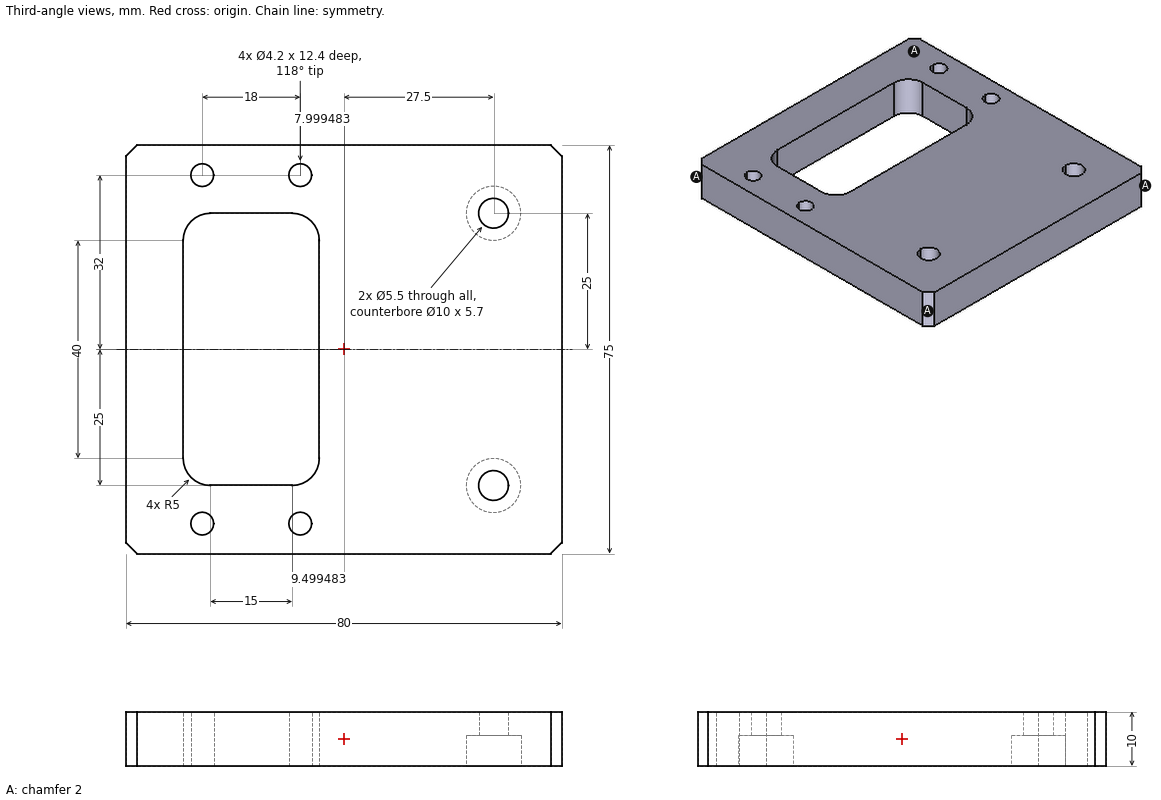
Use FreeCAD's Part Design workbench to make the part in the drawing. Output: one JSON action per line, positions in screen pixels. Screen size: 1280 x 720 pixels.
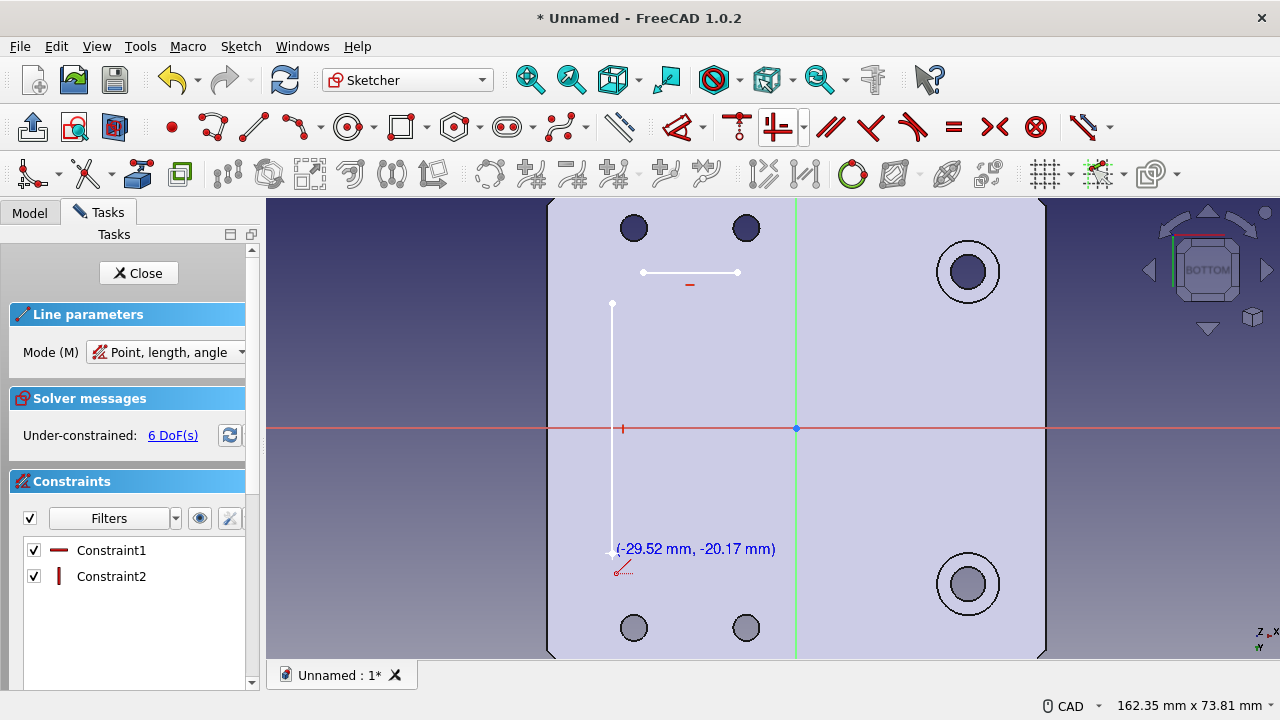
{"action": "left_click", "coordinate": [643, 584]}
{"action": "left_click", "coordinate": [737, 584]}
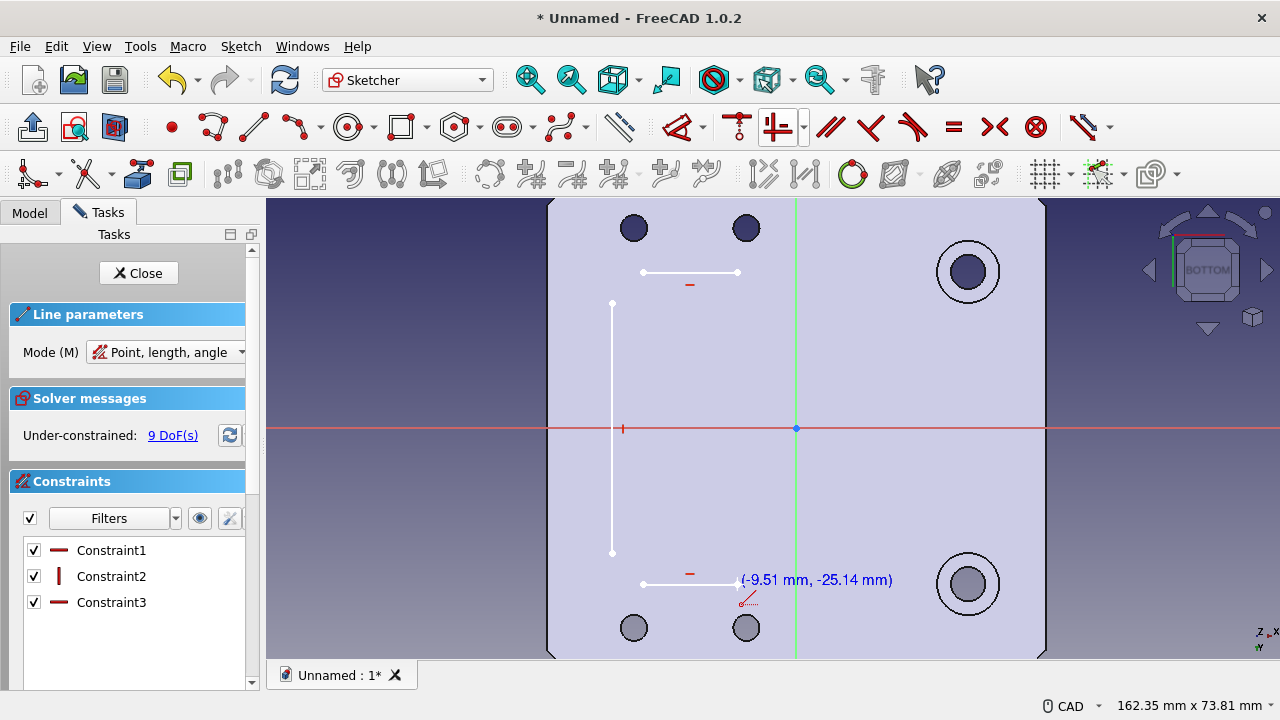
{"action": "left_click", "coordinate": [768, 553]}
{"action": "left_click", "coordinate": [768, 303]}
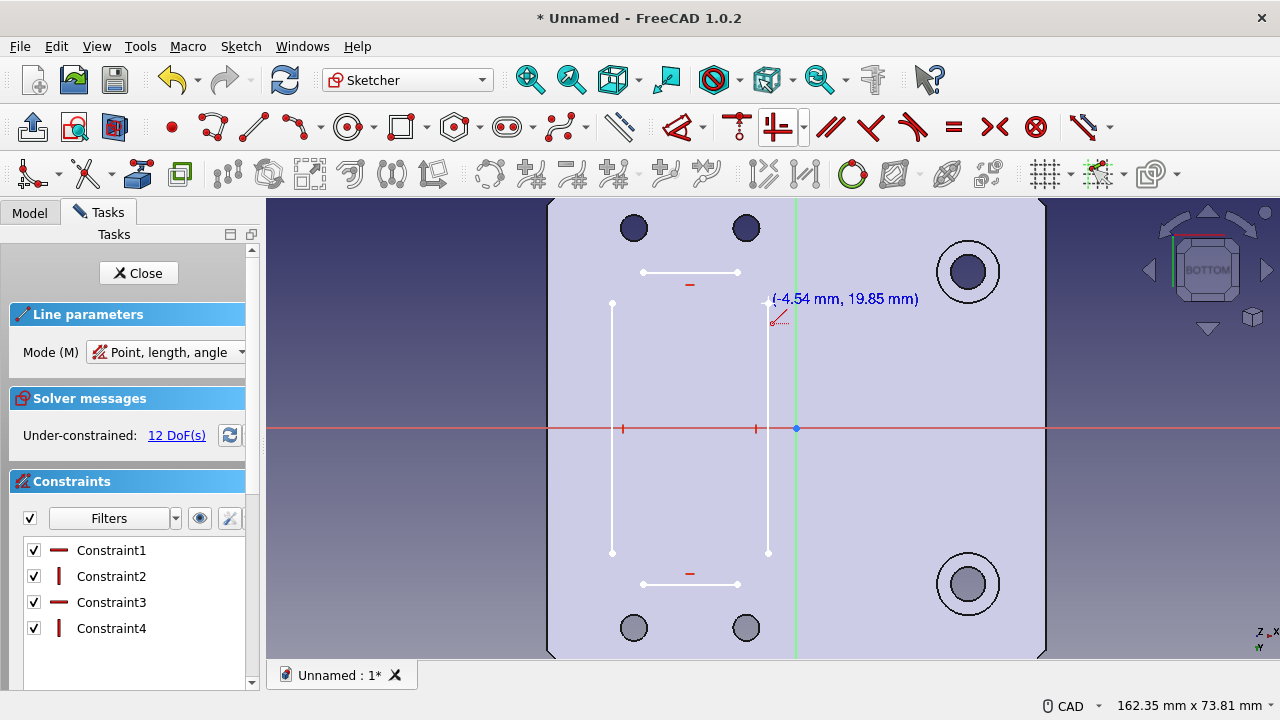
{"action": "key", "text": "g 3 a"}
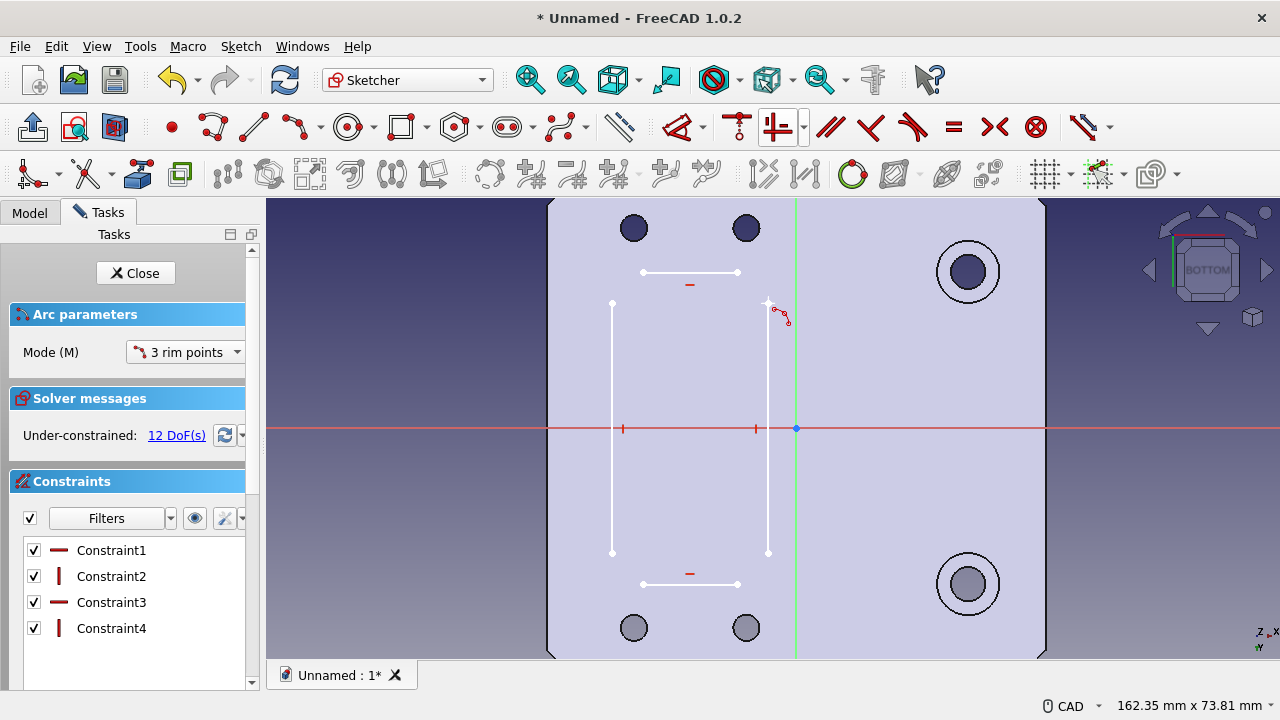
{"action": "left_click", "coordinate": [643, 273]}
{"action": "left_click", "coordinate": [612, 304]}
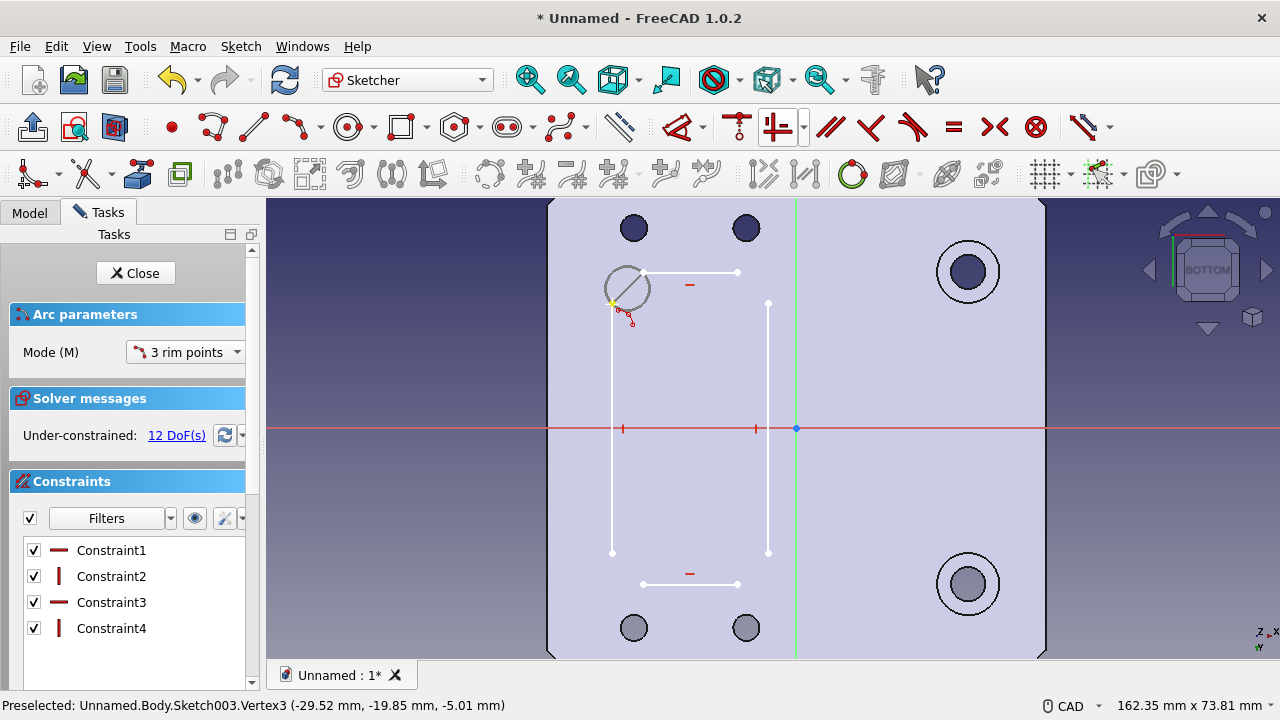
{"action": "scroll", "coordinate": [621, 281], "scroll_direction": "up", "scroll_amount": 3}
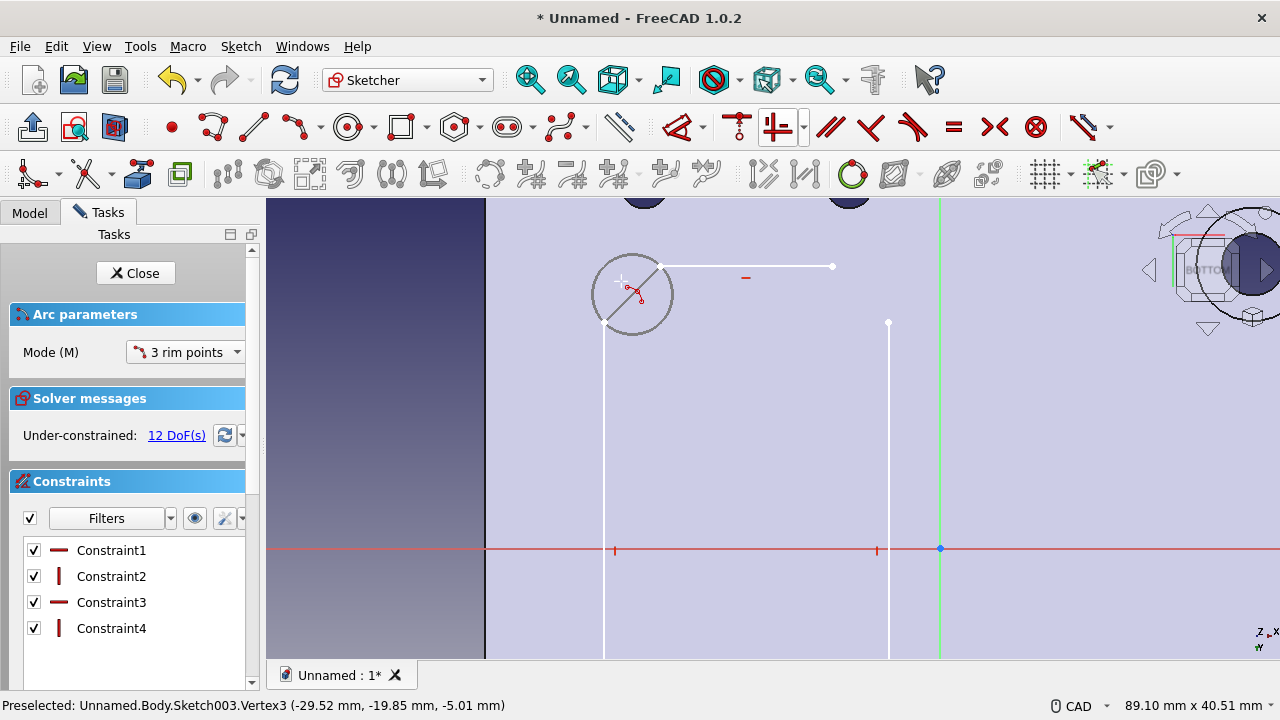
{"action": "left_click", "coordinate": [621, 281]}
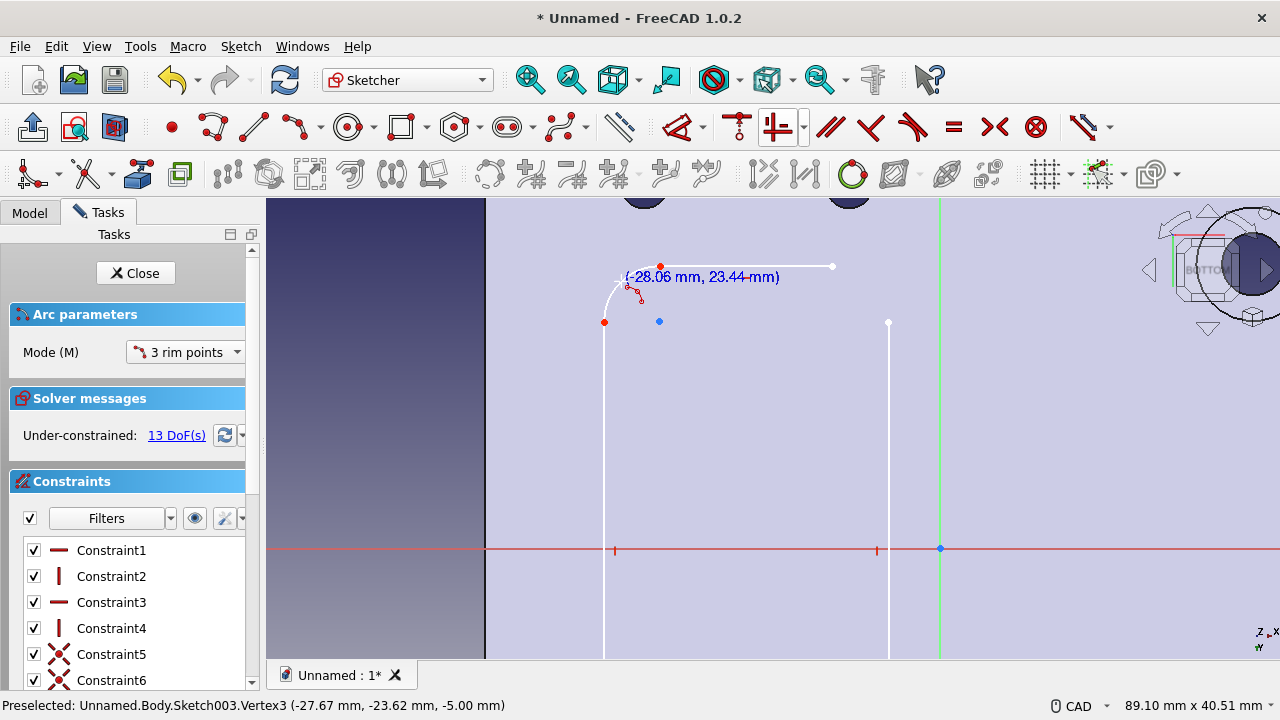
{"action": "scroll", "coordinate": [622, 282], "scroll_direction": "down", "scroll_amount": 3}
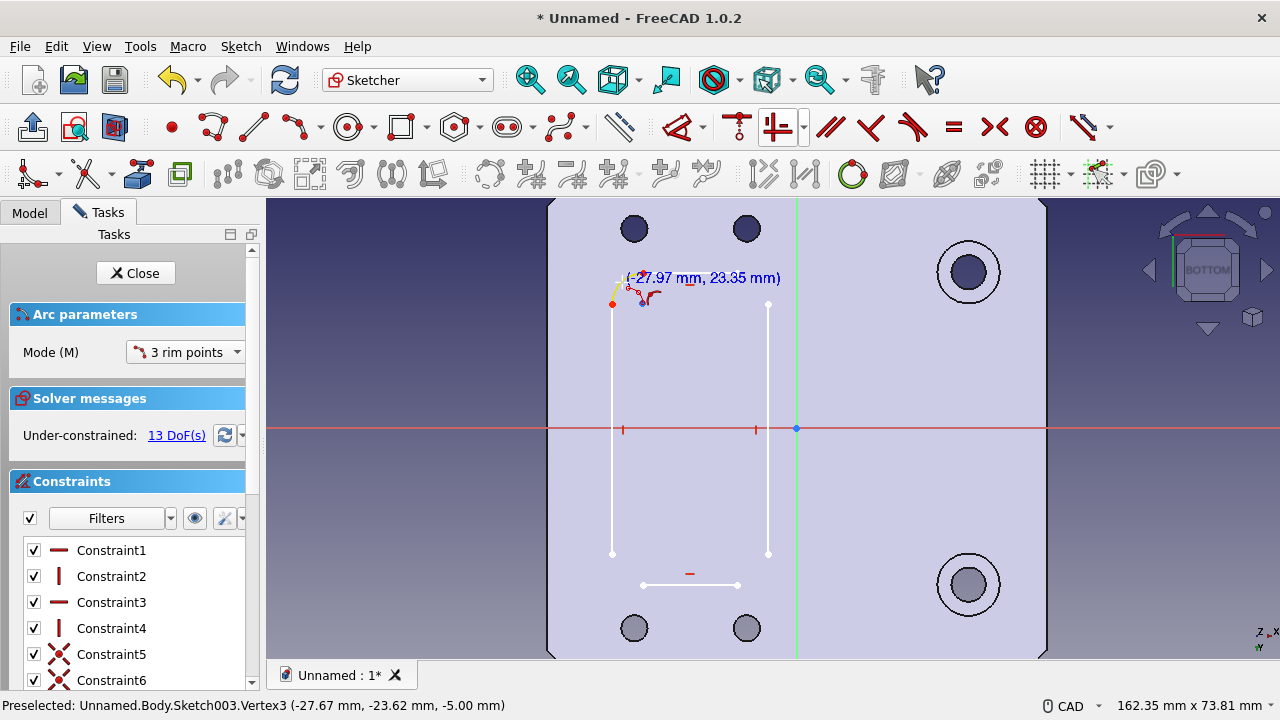
{"action": "left_click", "coordinate": [612, 554]}
{"action": "left_click", "coordinate": [643, 585]}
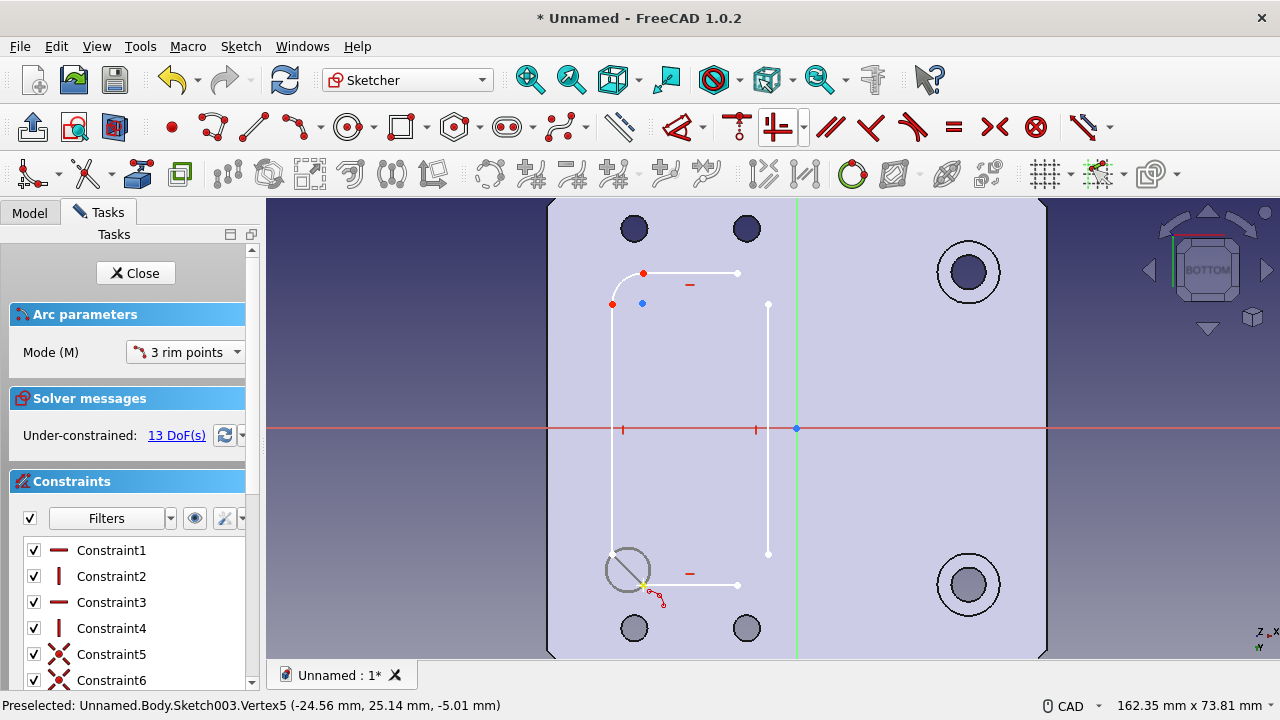
{"action": "scroll", "coordinate": [622, 575], "scroll_direction": "up", "scroll_amount": 3}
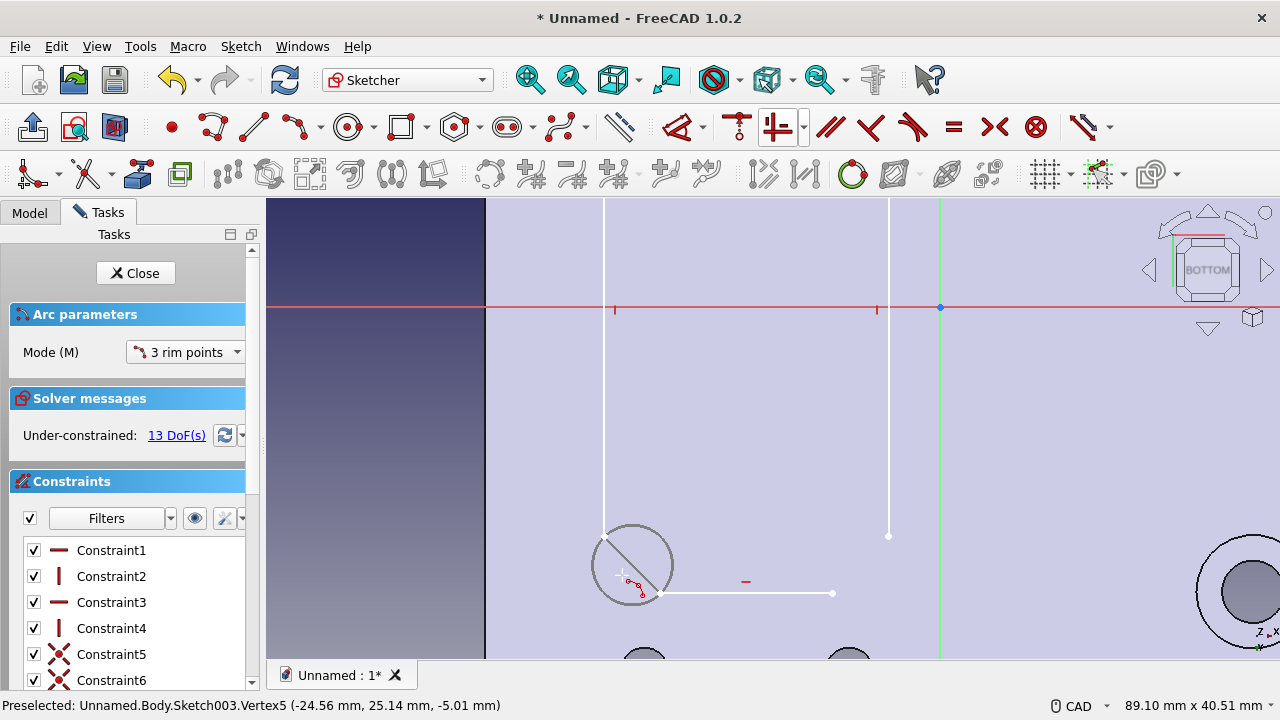
{"action": "left_click", "coordinate": [621, 575]}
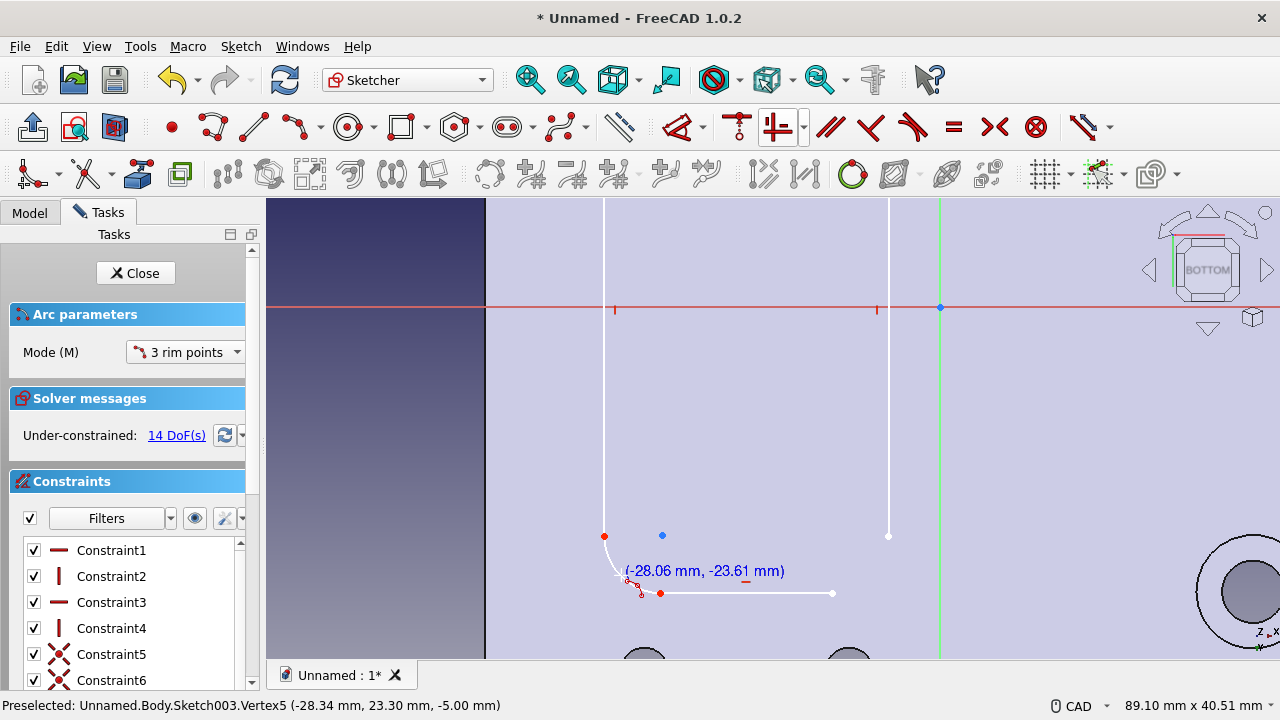
{"action": "left_click", "coordinate": [832, 593]}
{"action": "left_click", "coordinate": [889, 537]}
{"action": "left_click", "coordinate": [872, 575]}